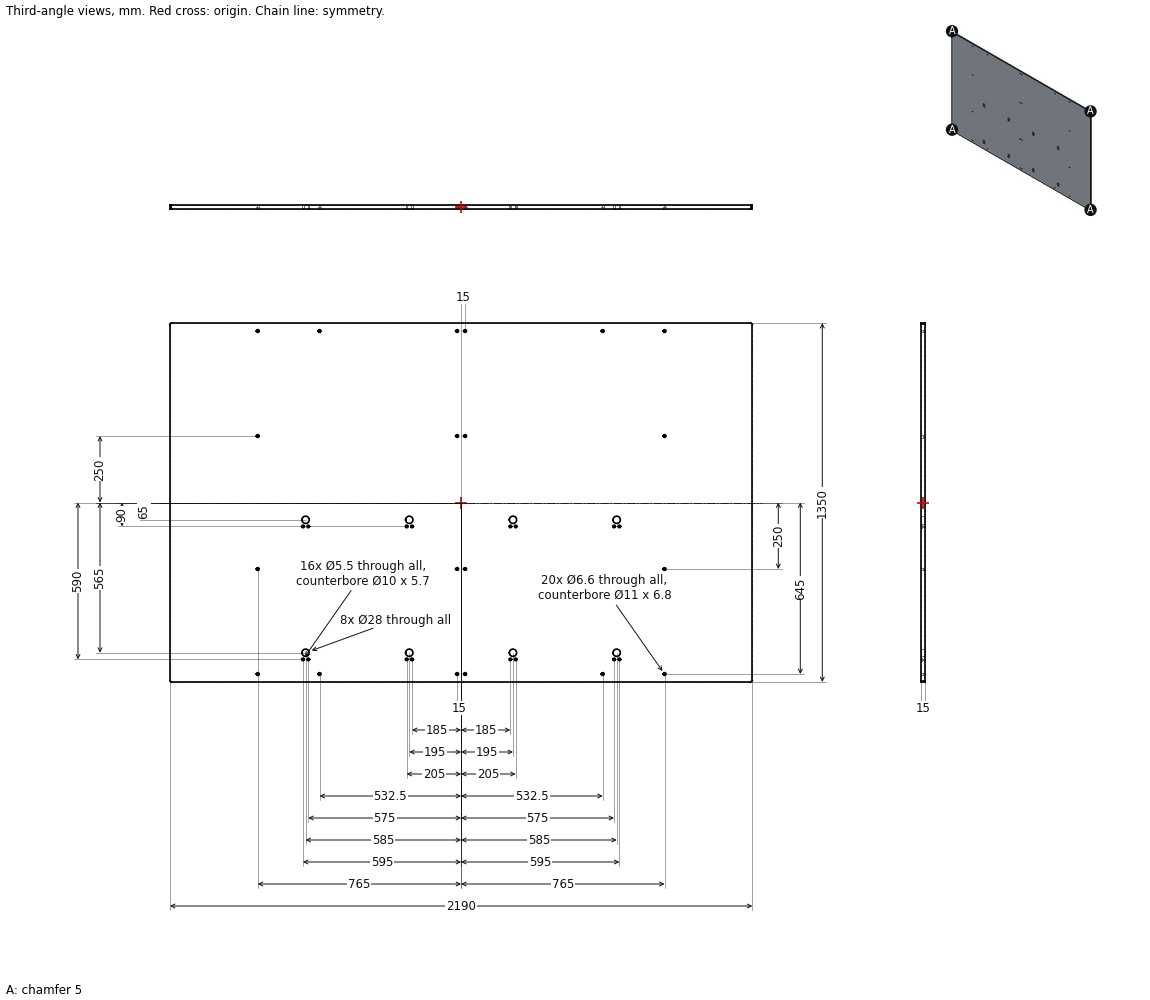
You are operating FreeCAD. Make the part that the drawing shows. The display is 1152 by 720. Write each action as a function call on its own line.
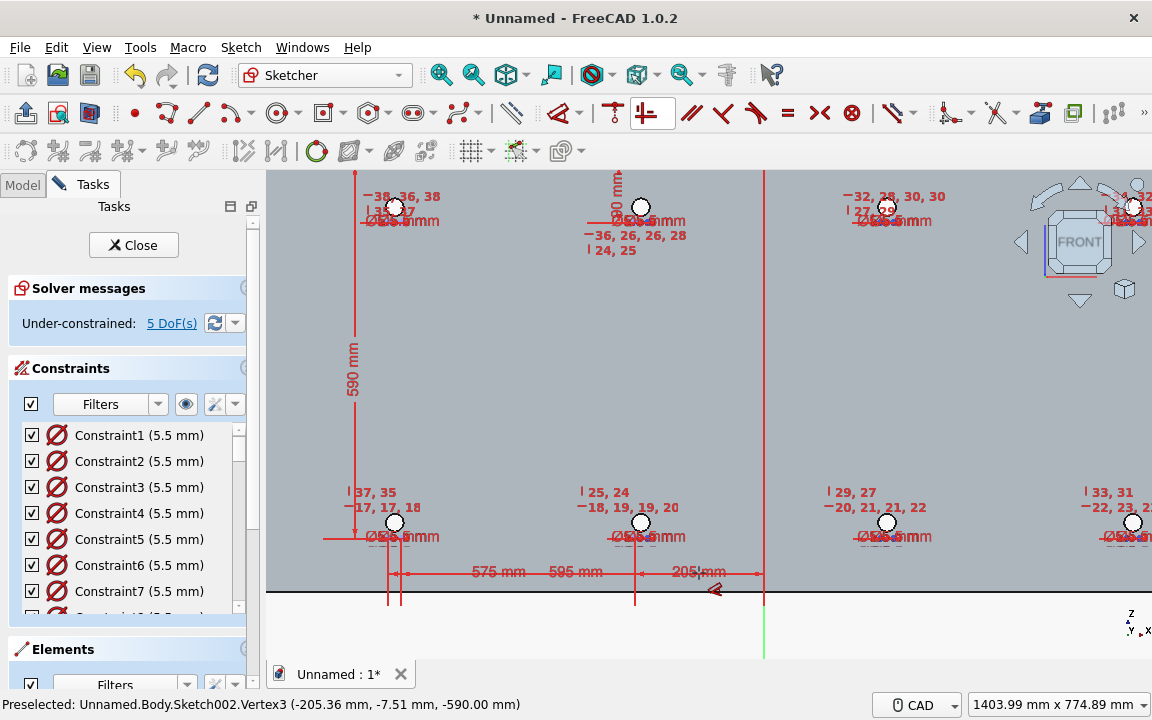
click(647, 539)
click(706, 597)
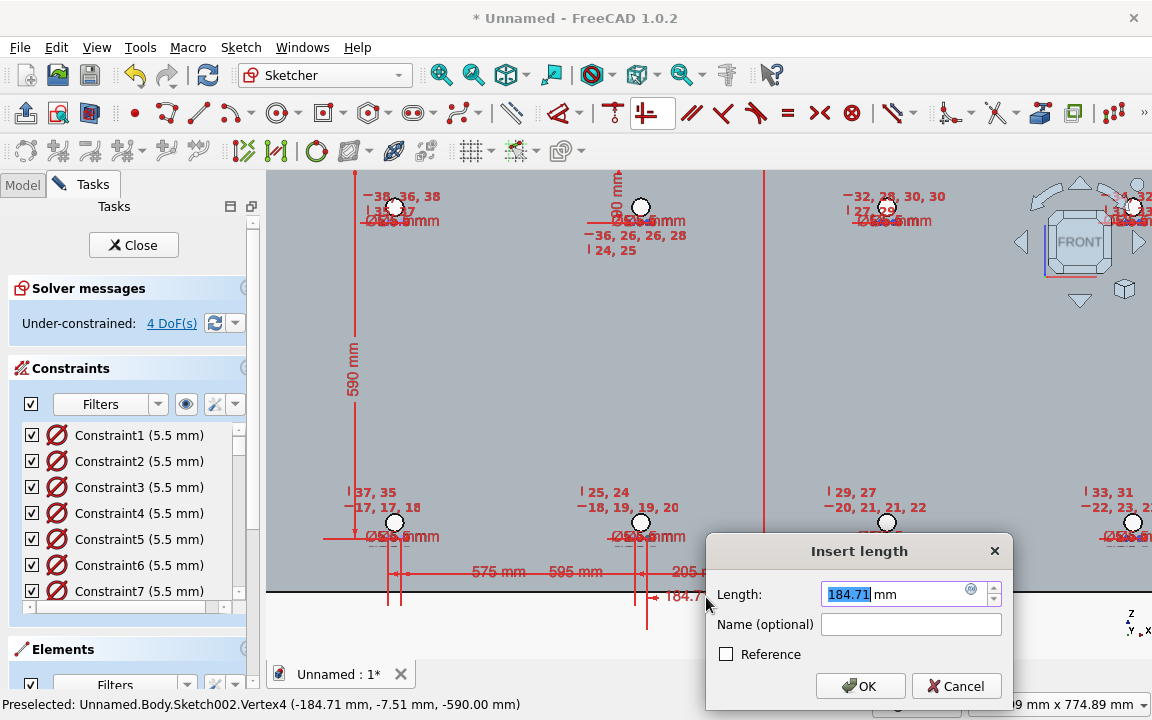
text(185)
key(Return)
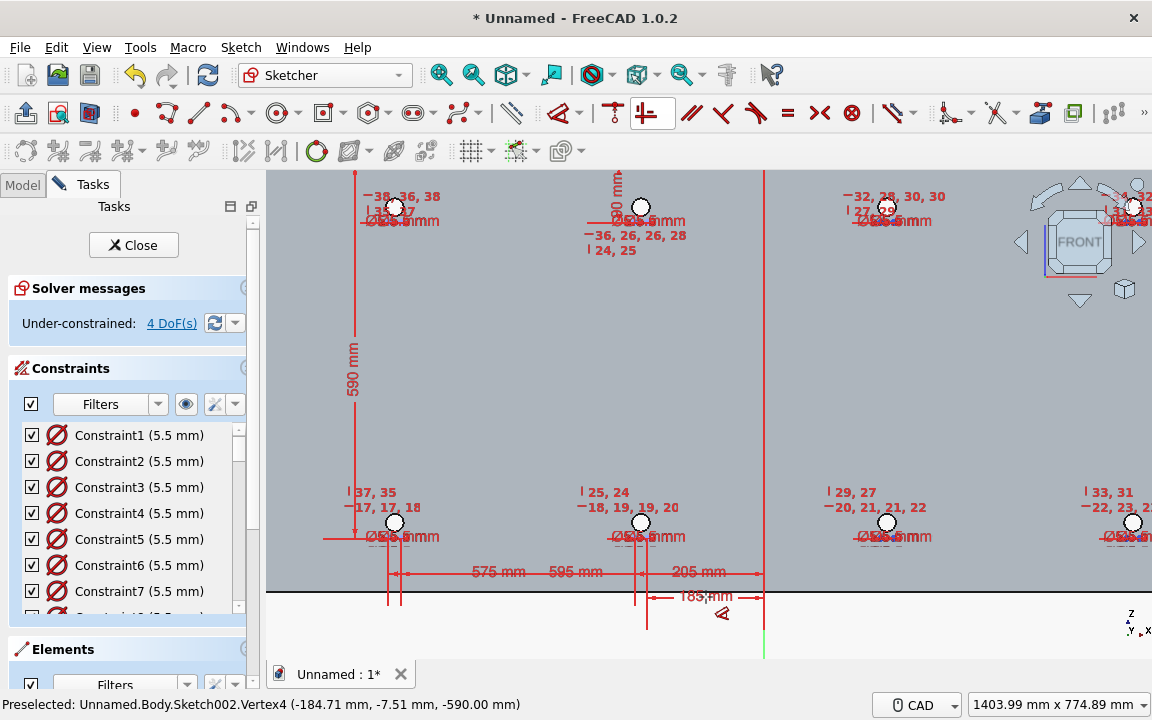
click(880, 539)
click(822, 573)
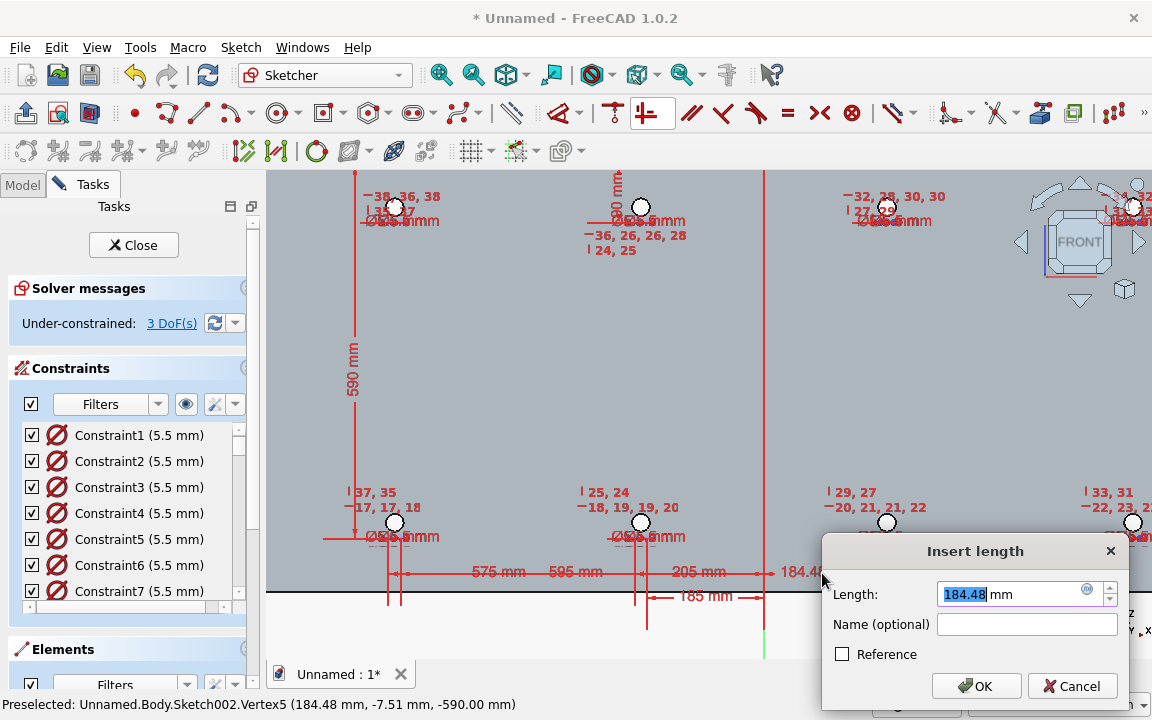
text(185)
key(Return)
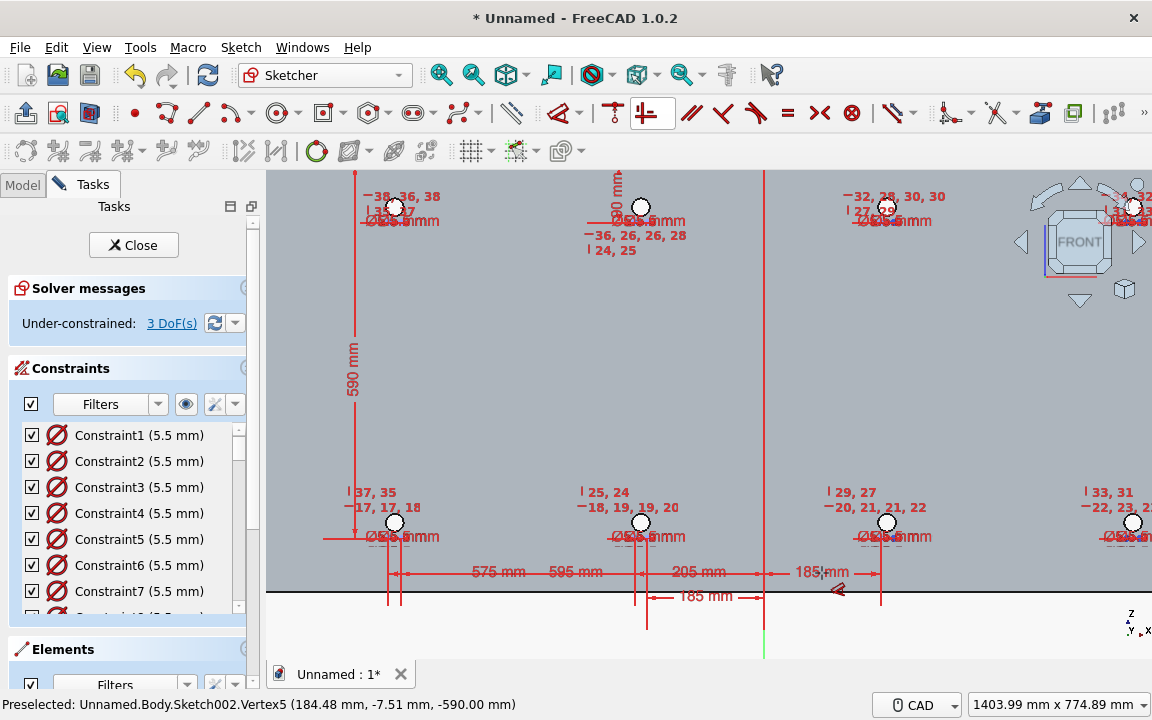
click(894, 539)
click(829, 597)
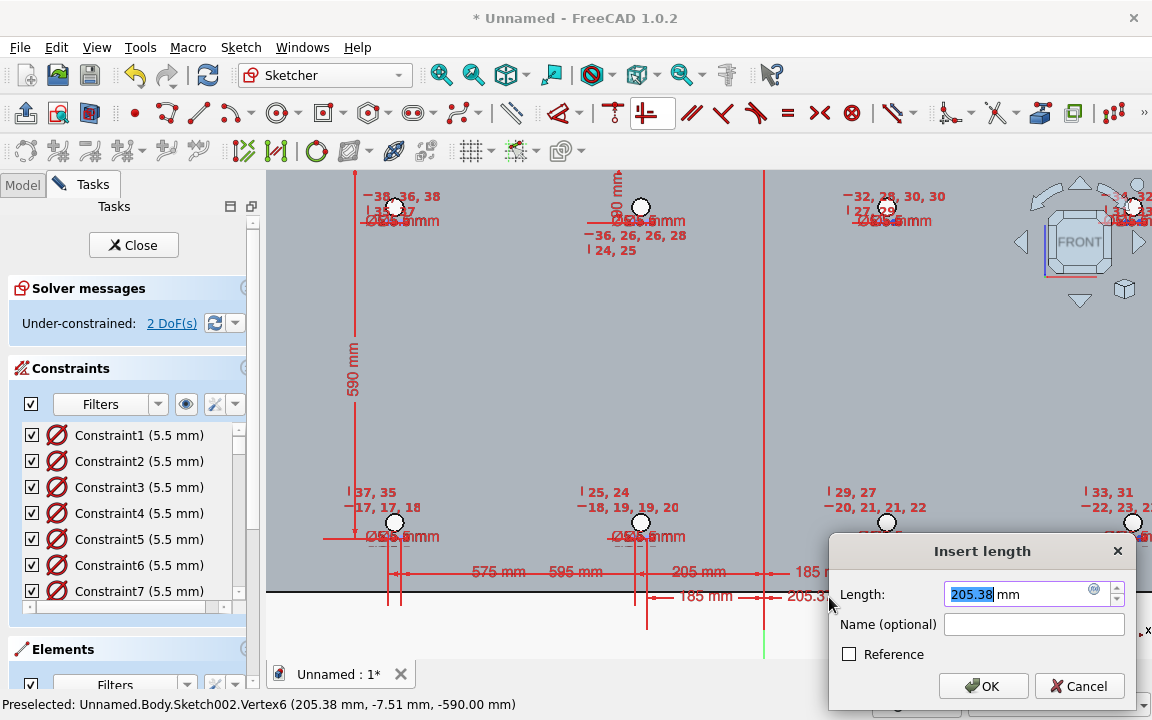
text(205)
key(Return)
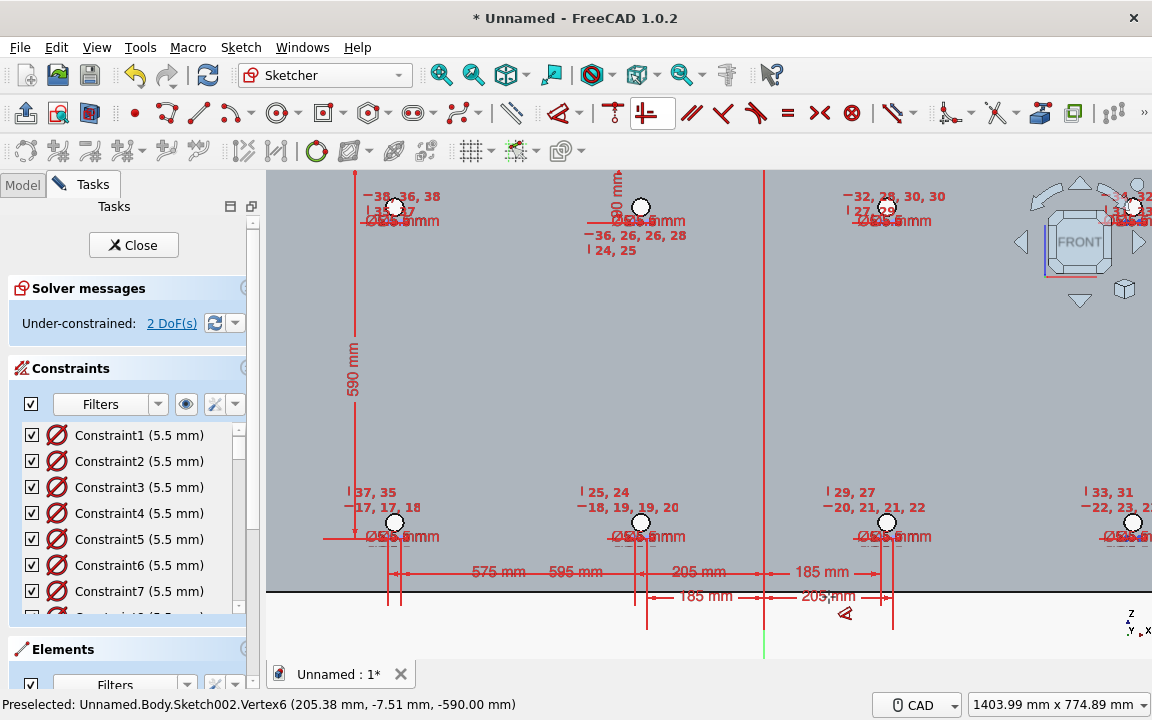
scroll(389, 539, down, 2)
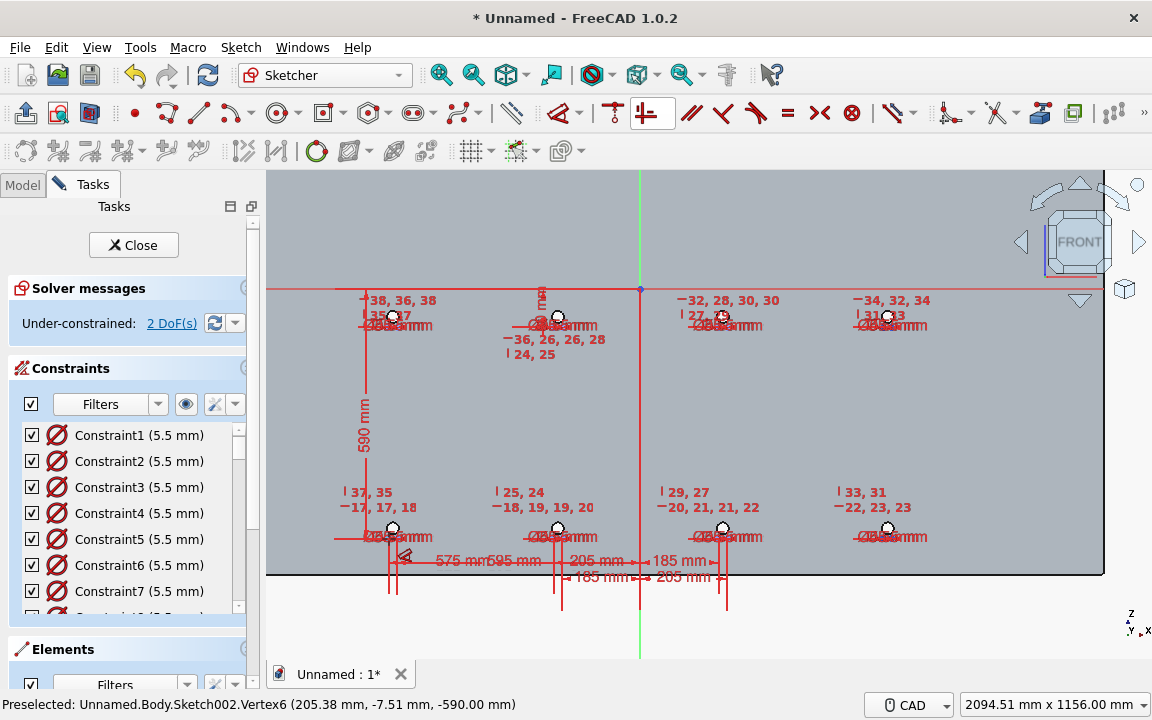
scroll(883, 539, up, 2)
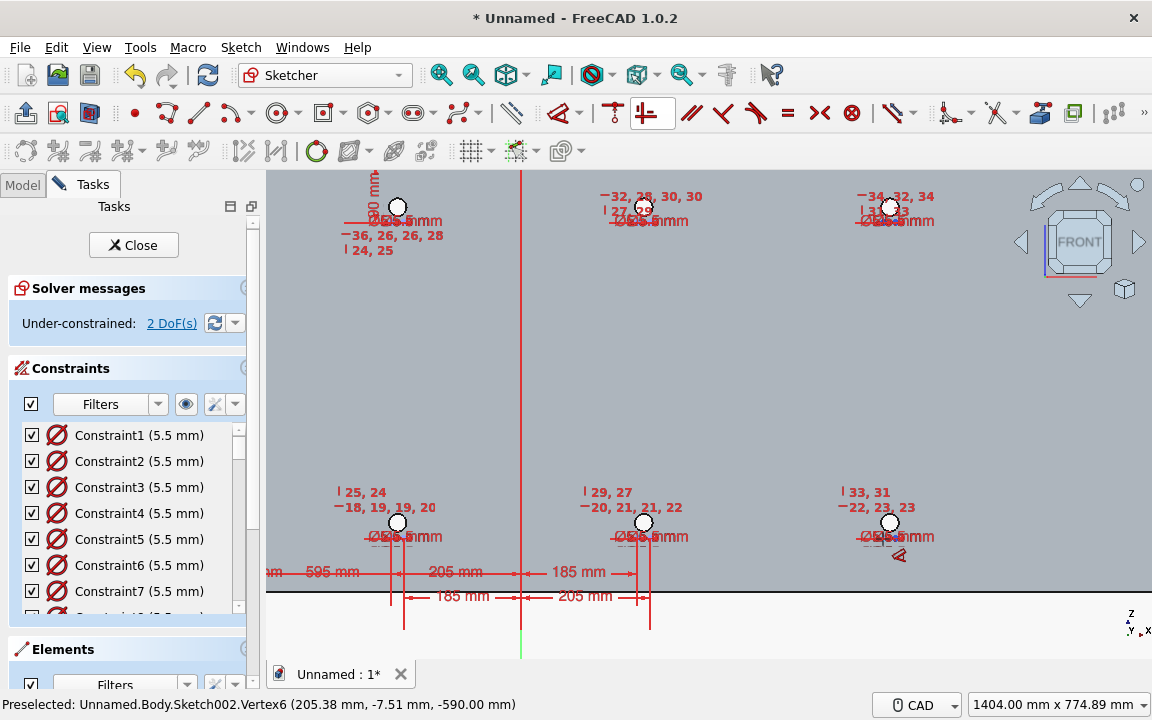
click(883, 539)
click(702, 573)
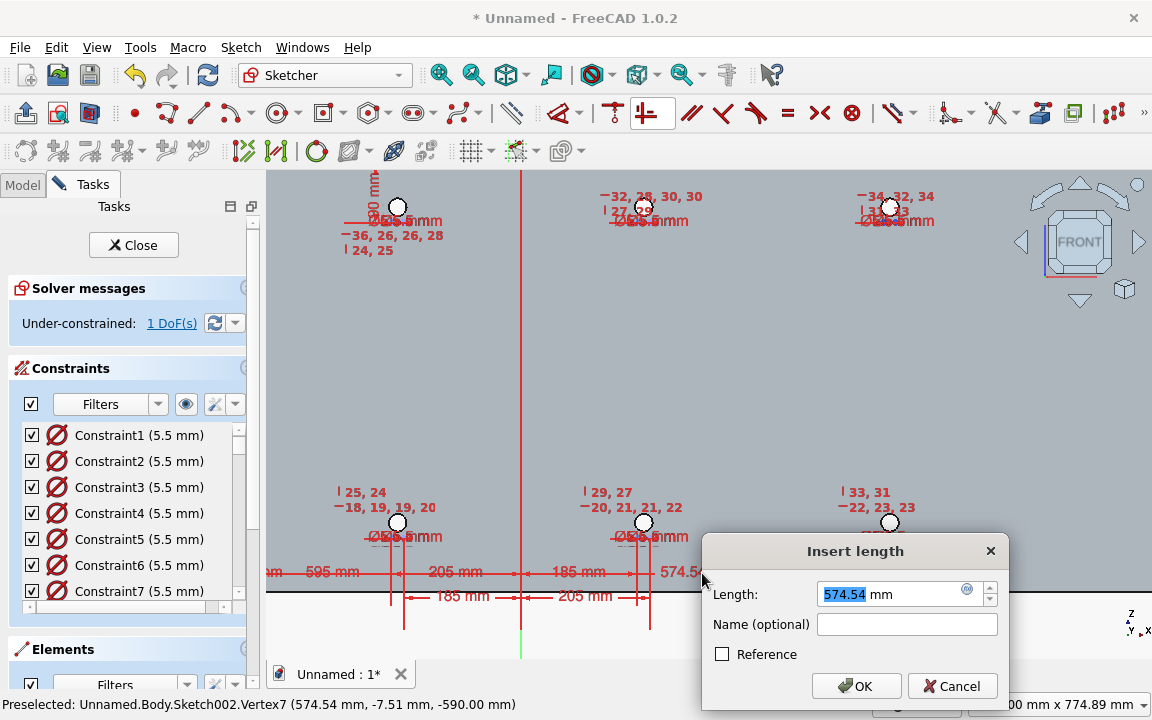
text(575)
key(Return)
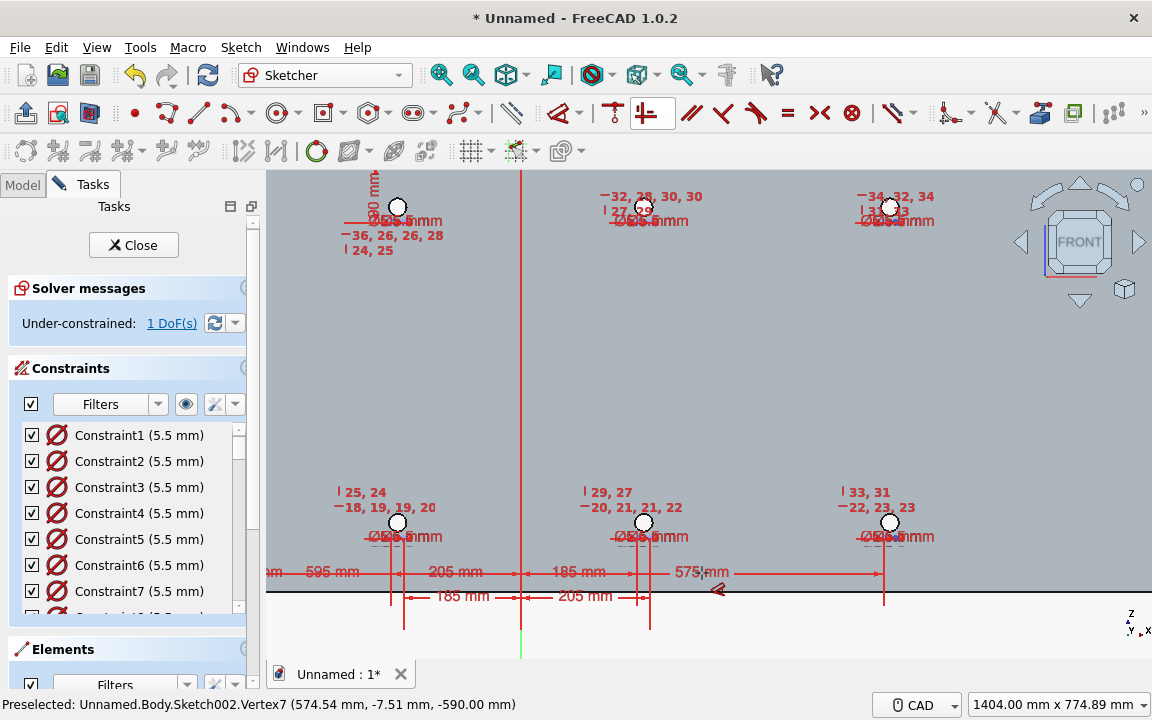
click(896, 539)
click(795, 573)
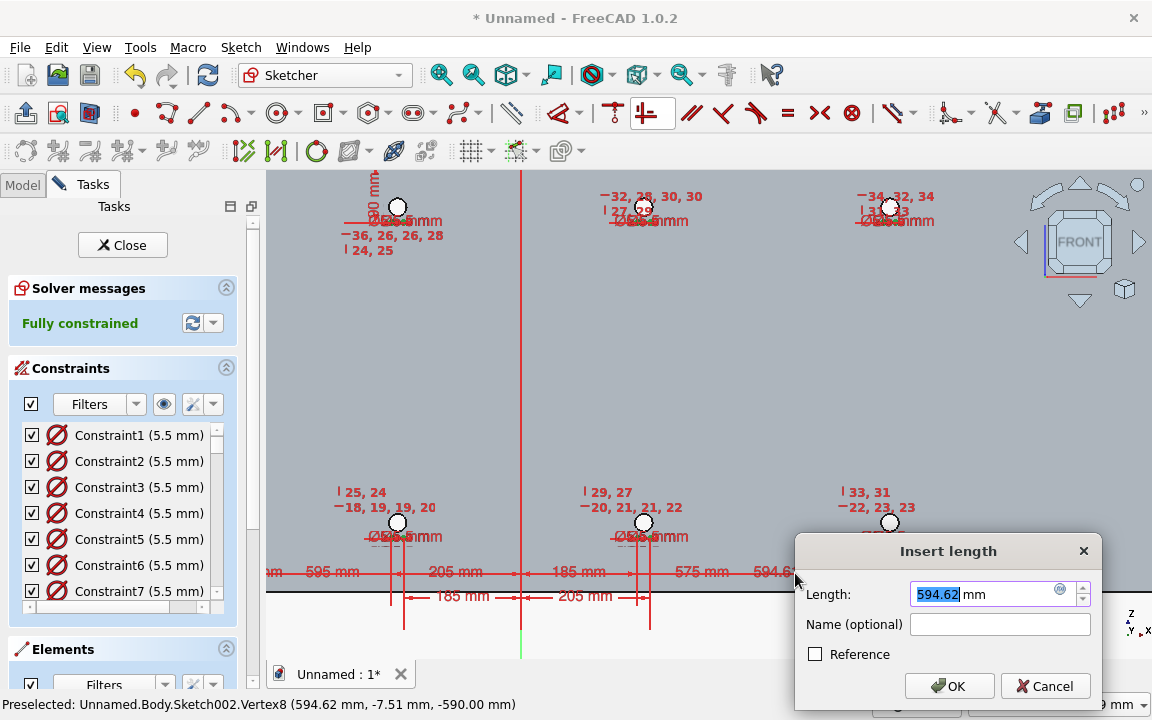
text(595)
key(Return)
key(Escape)